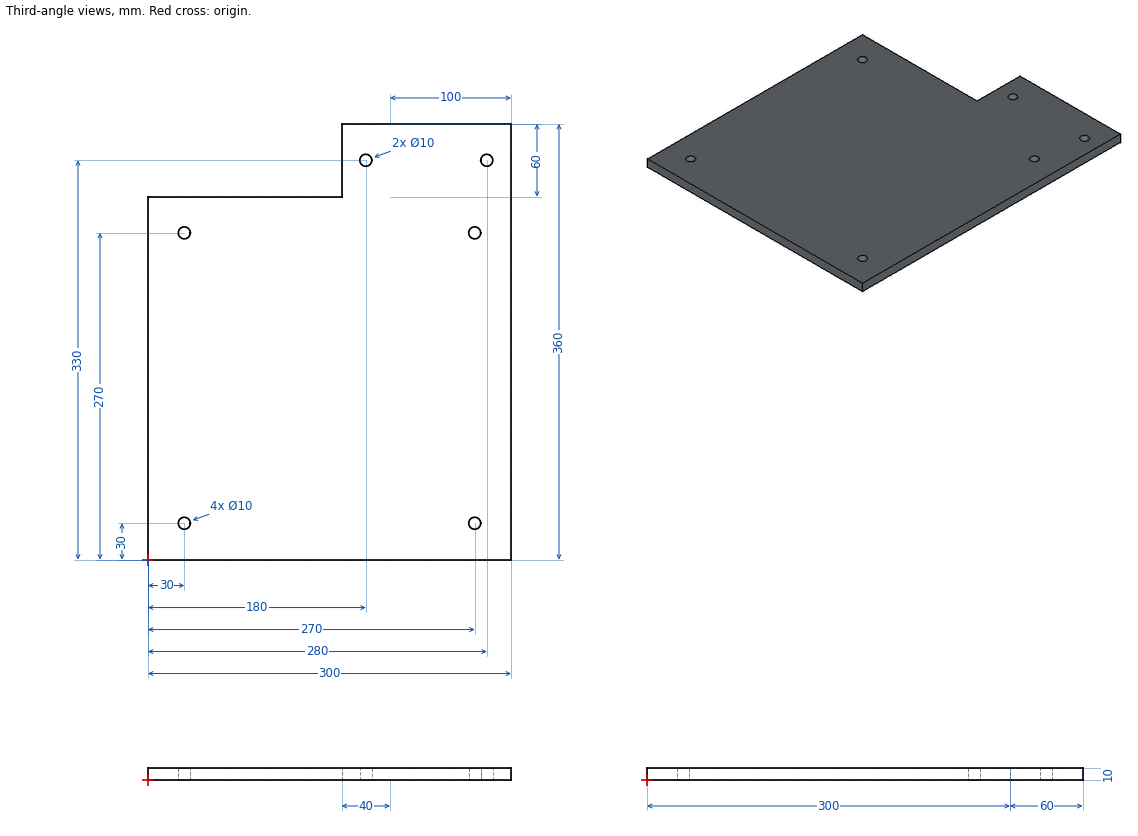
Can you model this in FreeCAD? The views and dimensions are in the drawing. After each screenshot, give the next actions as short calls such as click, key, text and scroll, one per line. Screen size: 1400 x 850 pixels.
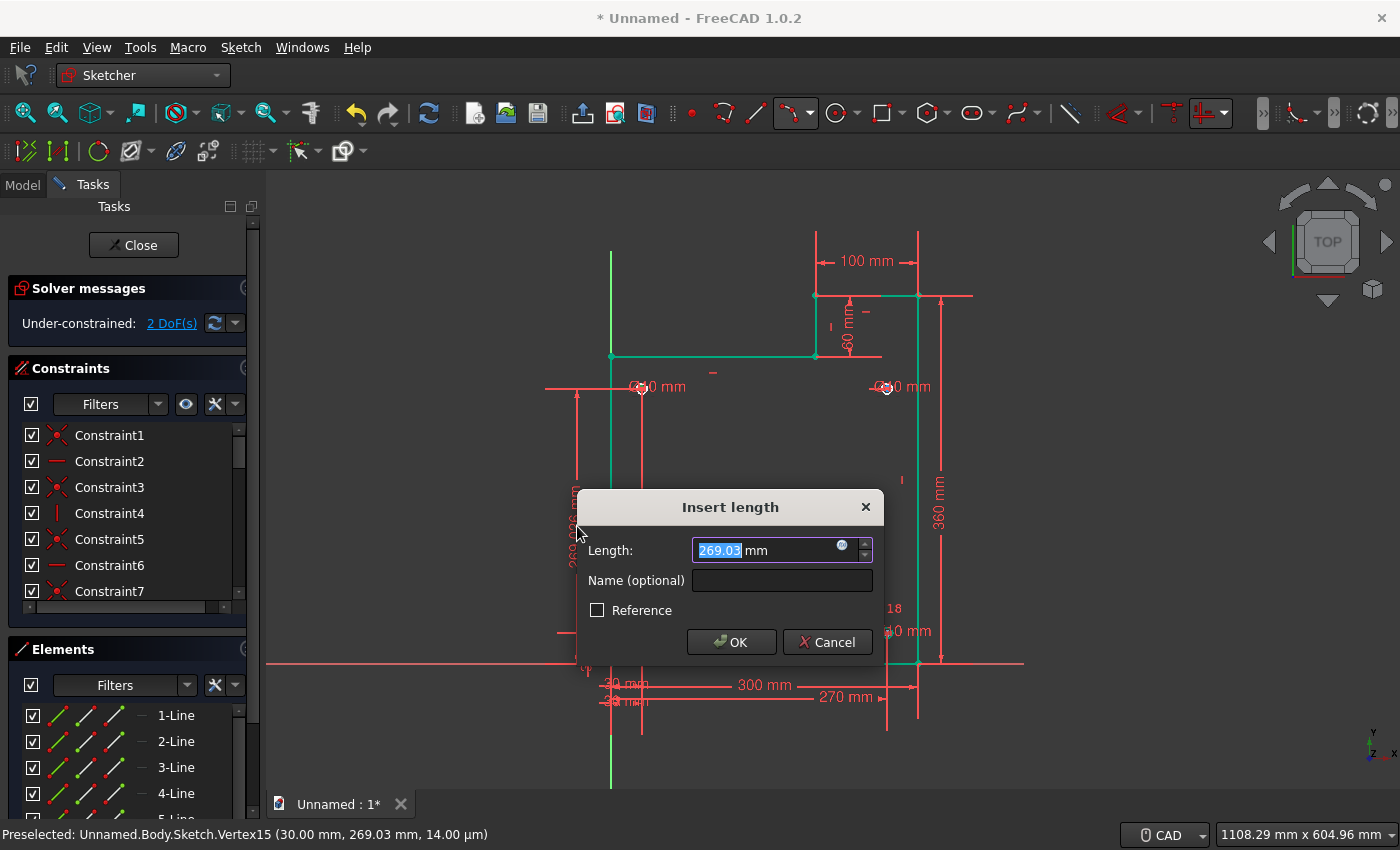
text(270)
key(Return)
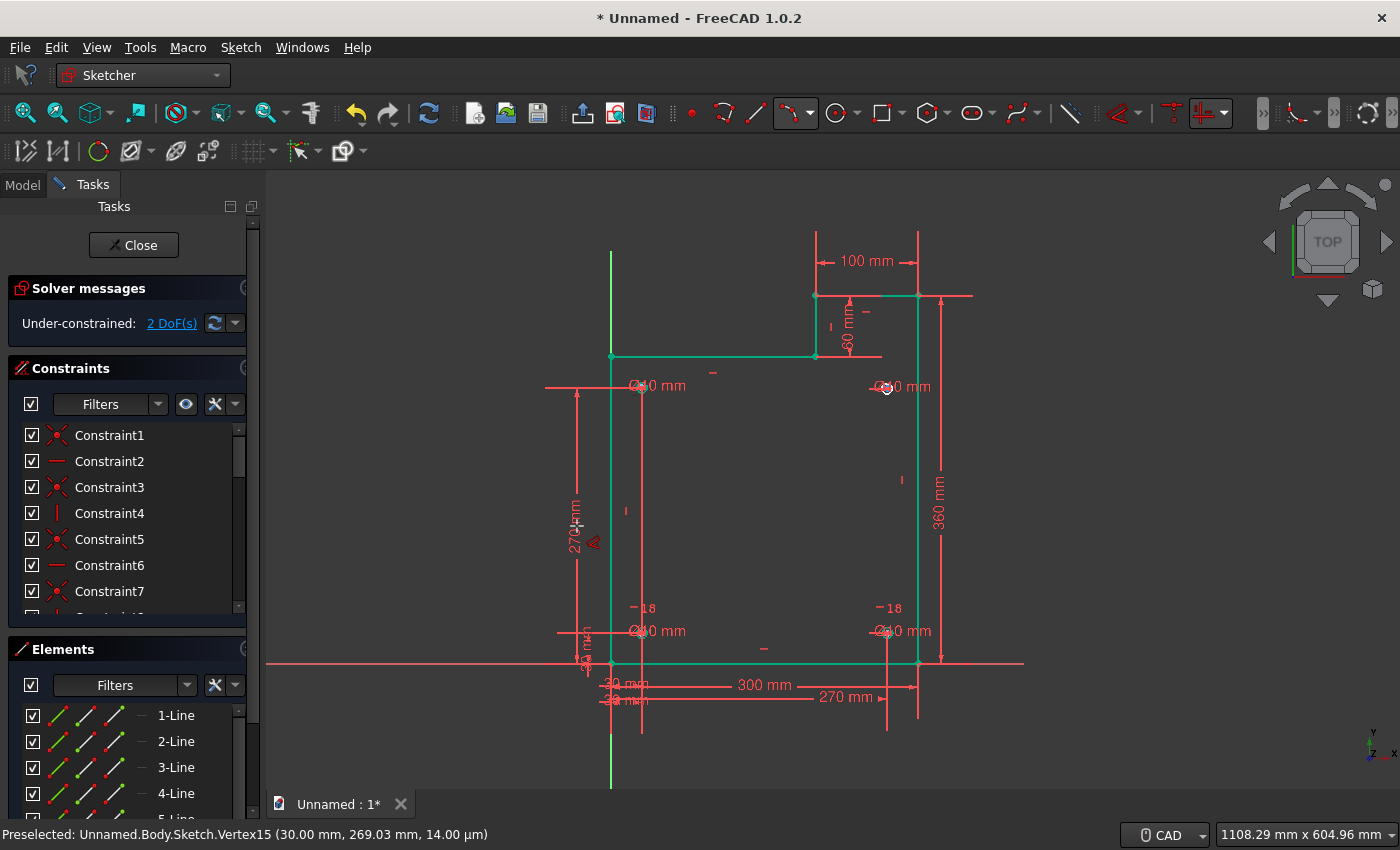
click(887, 389)
click(846, 355)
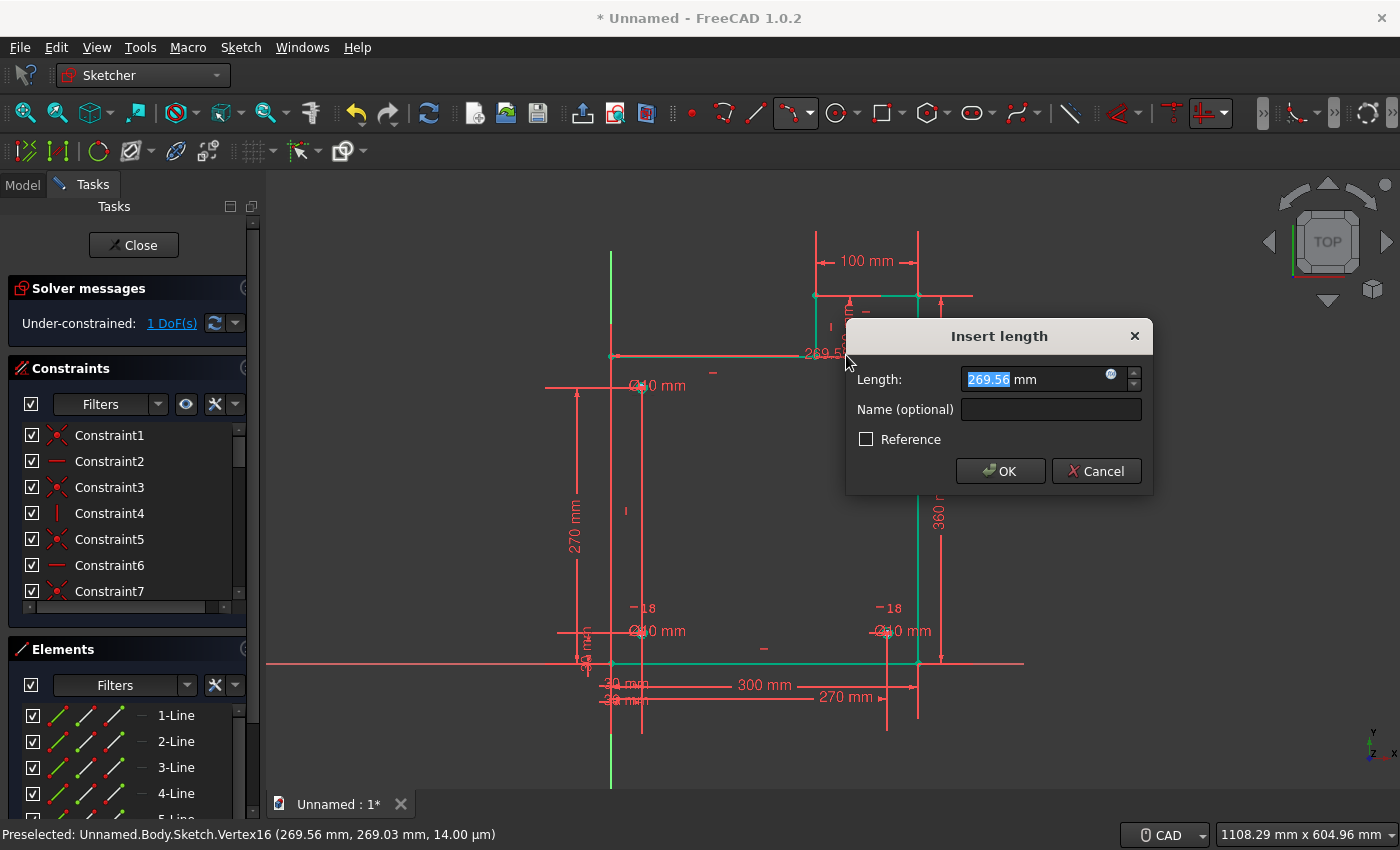
text(270)
key(Return)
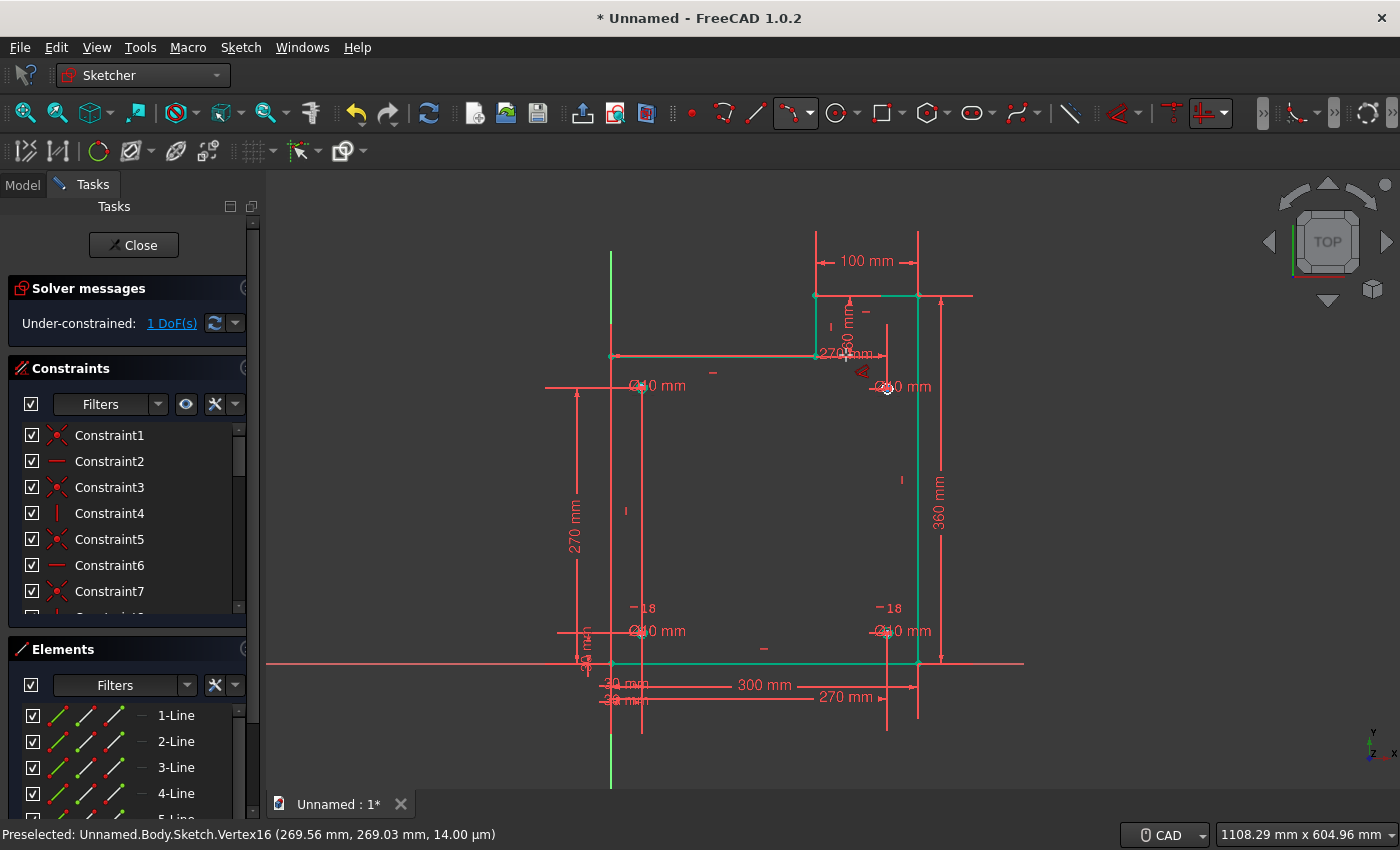
click(887, 389)
click(577, 463)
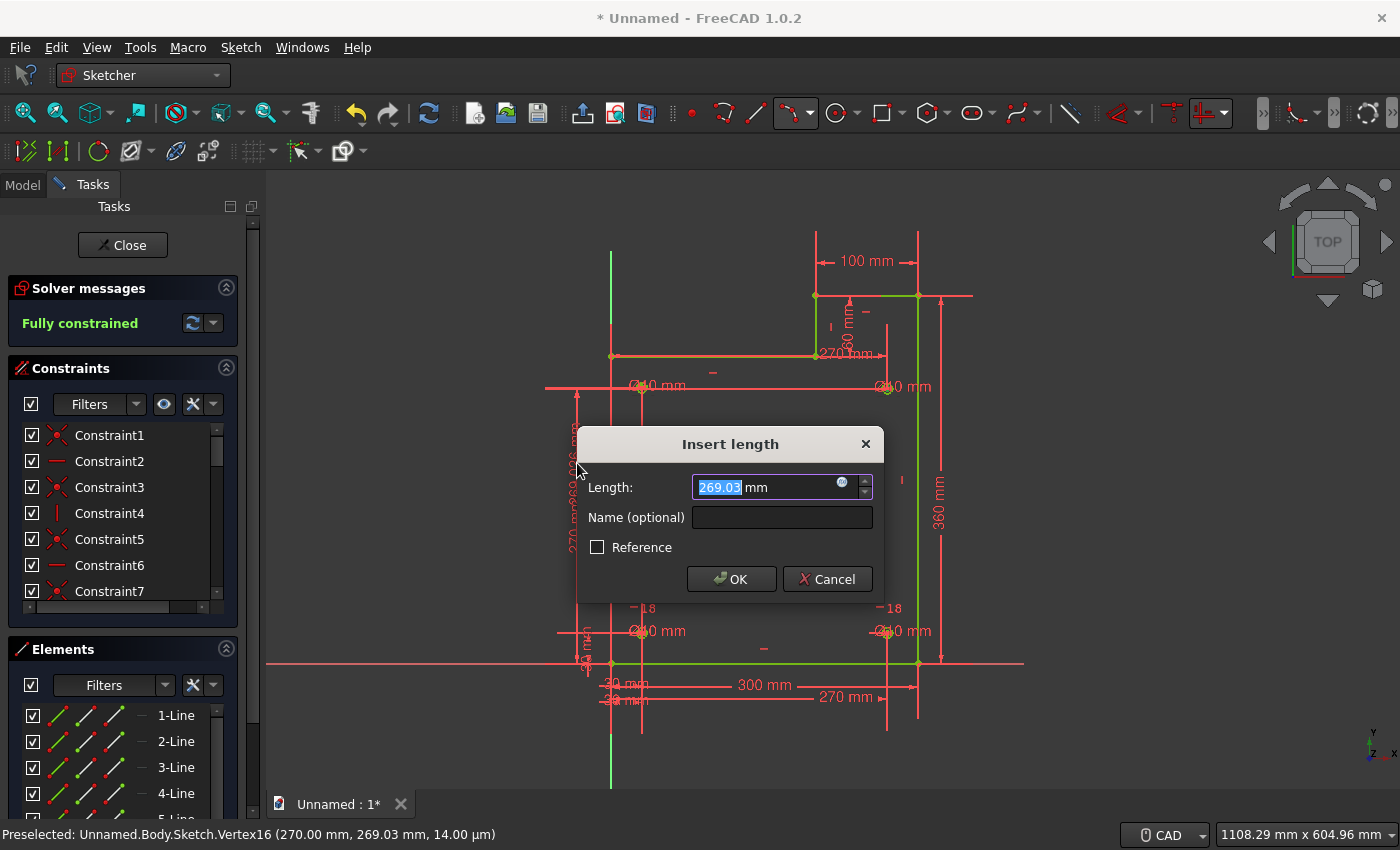
text(270)
key(Return)
key(Escape)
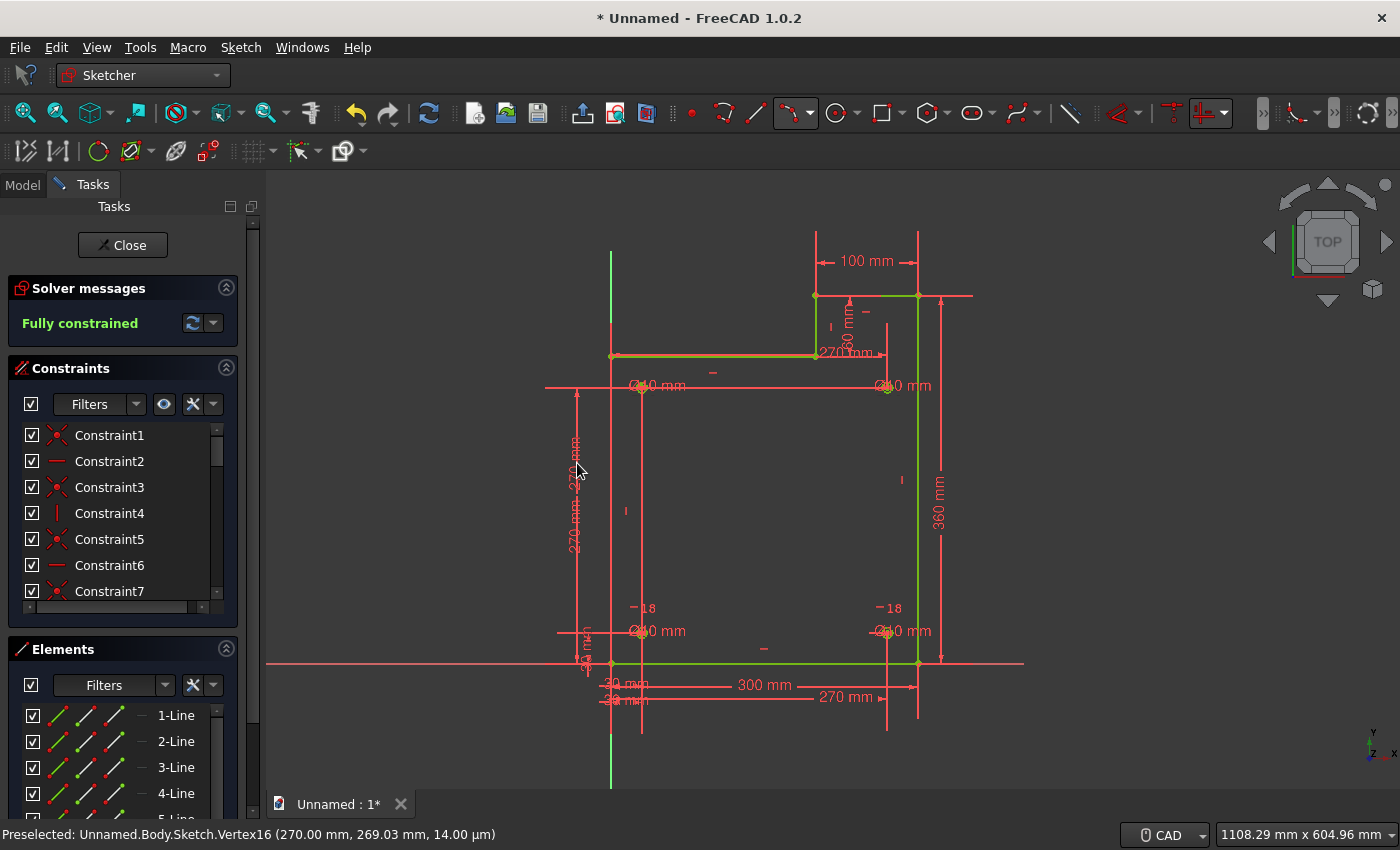
click(123, 245)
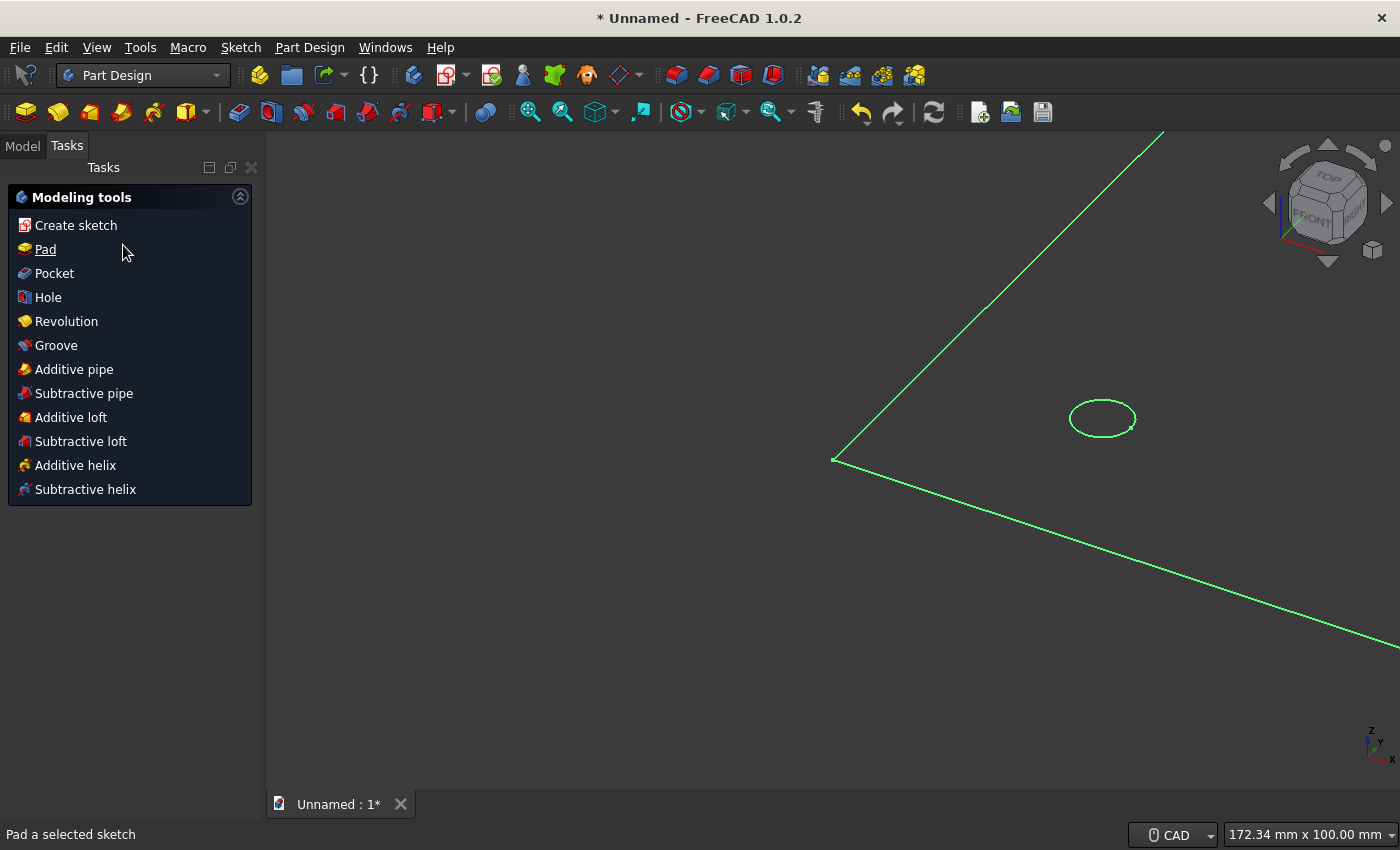
click(26, 112)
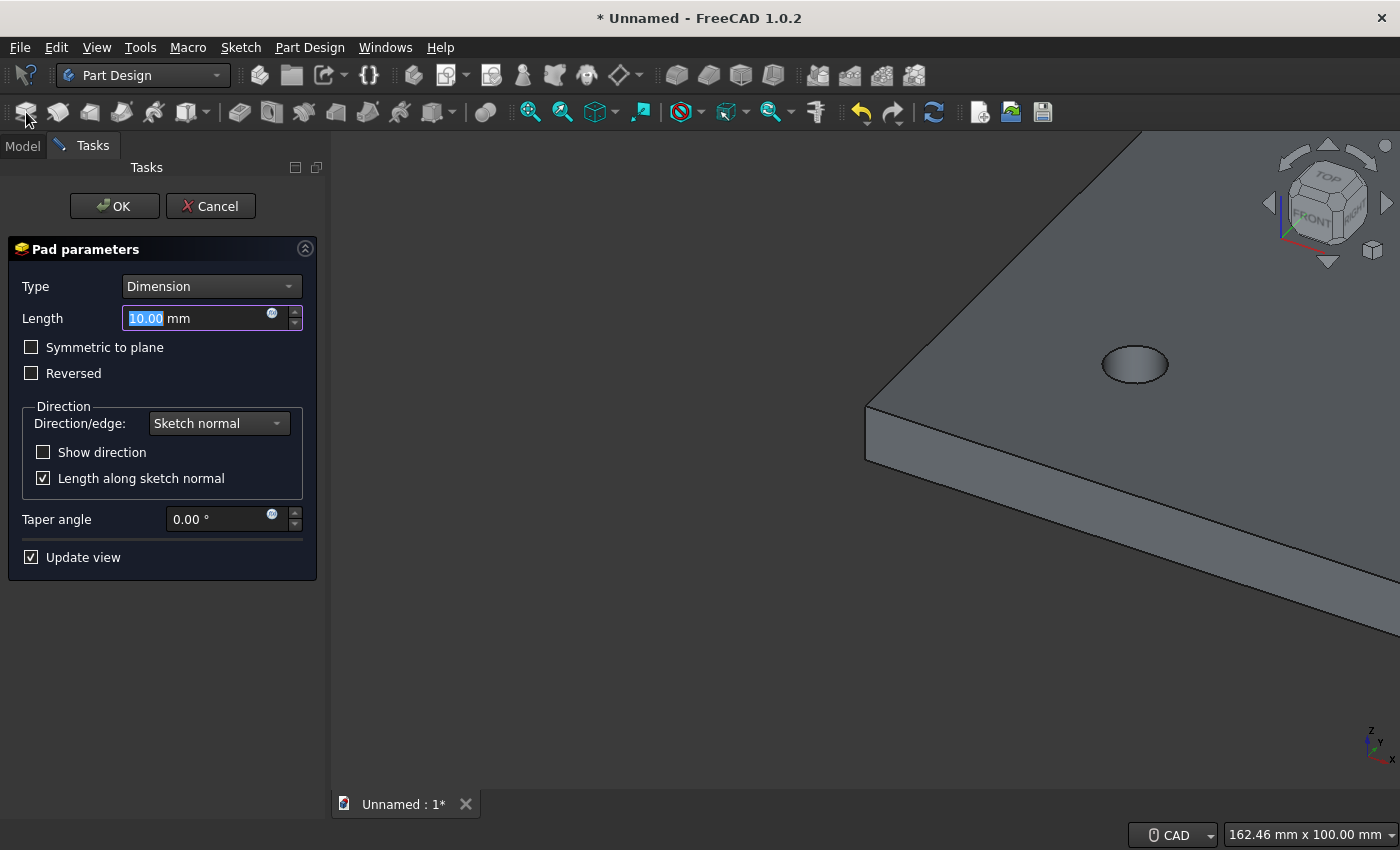
text(10)
key(Tab)